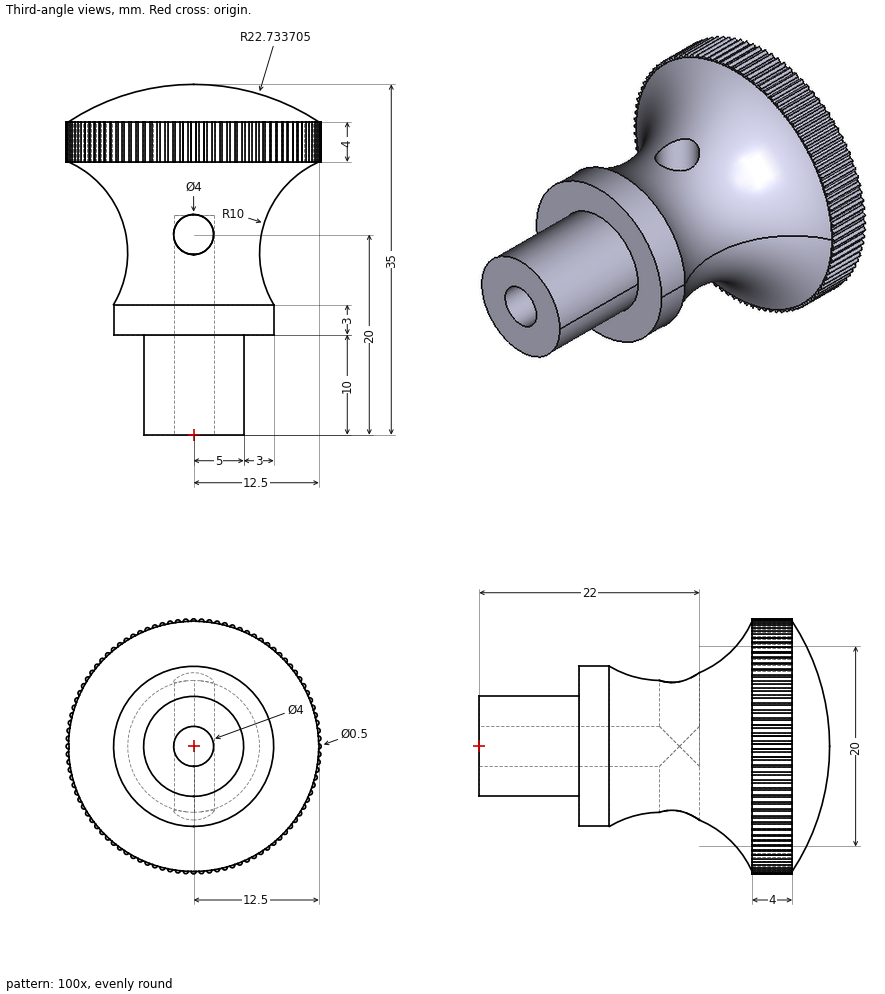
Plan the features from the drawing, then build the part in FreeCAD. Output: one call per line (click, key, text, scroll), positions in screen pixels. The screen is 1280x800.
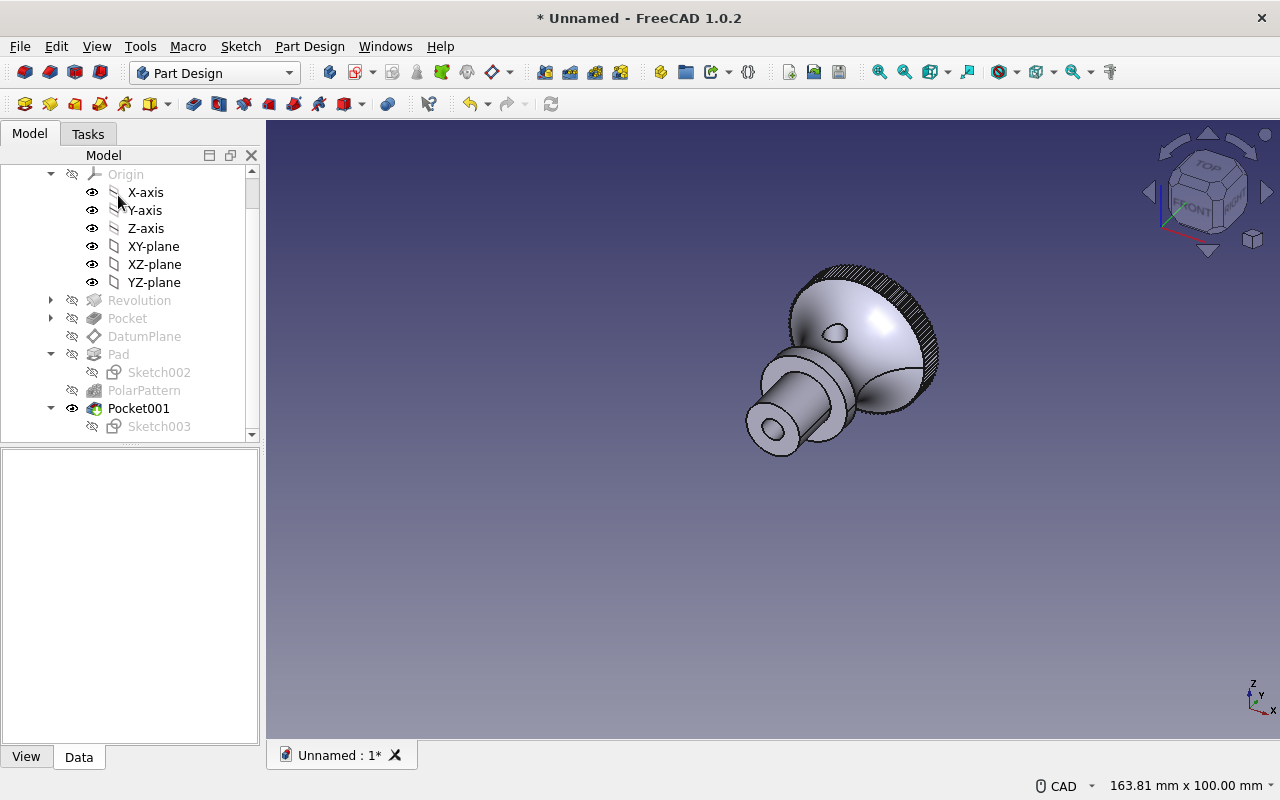
key(0)